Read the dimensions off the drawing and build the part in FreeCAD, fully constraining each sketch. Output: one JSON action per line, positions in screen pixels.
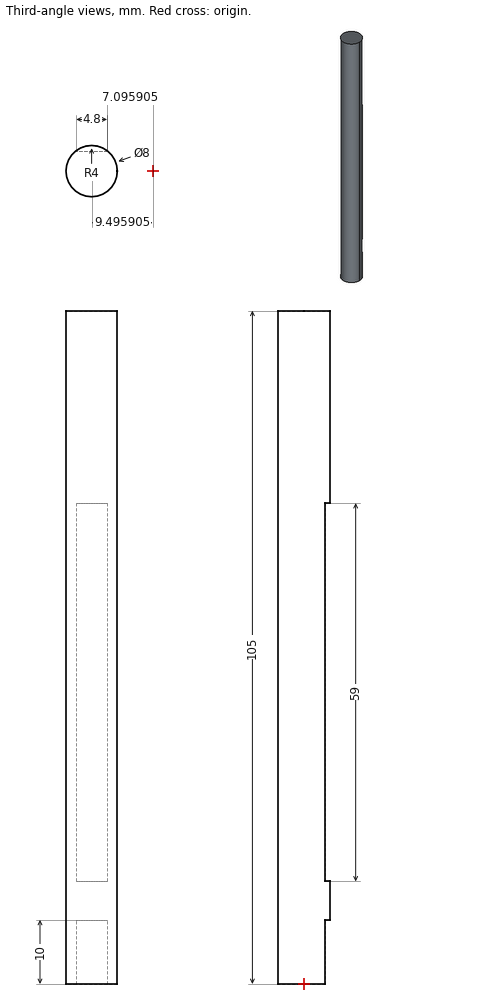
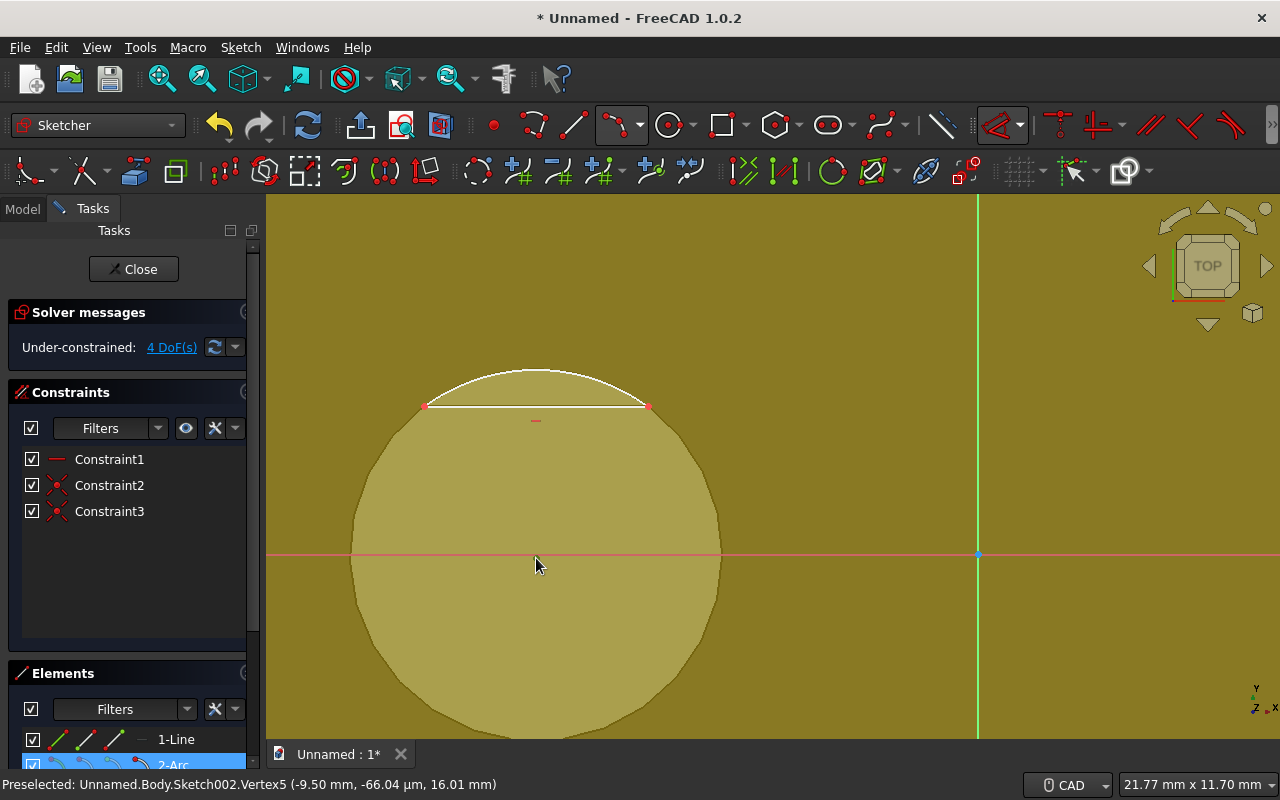
{"action": "left_click", "coordinate": [353, 555]}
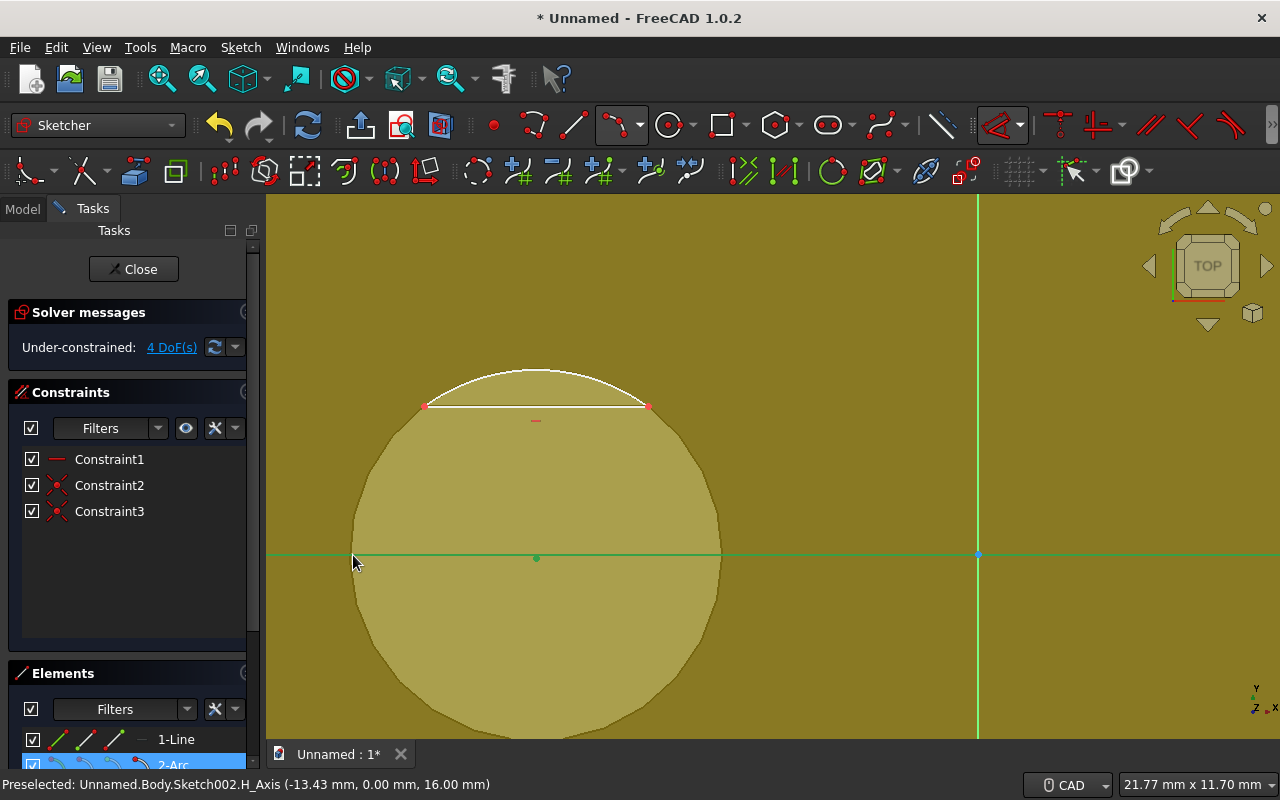
{"action": "key", "text": "c"}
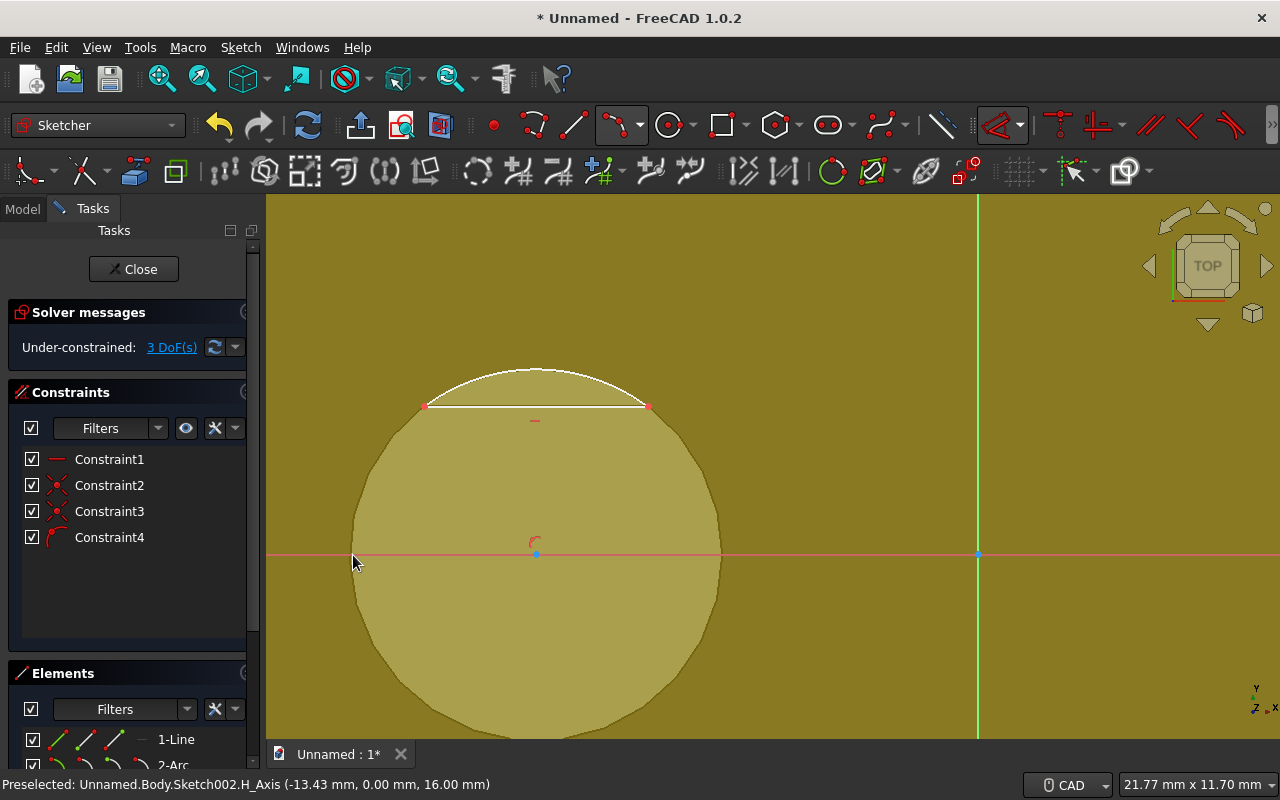
{"action": "left_click", "coordinate": [584, 376]}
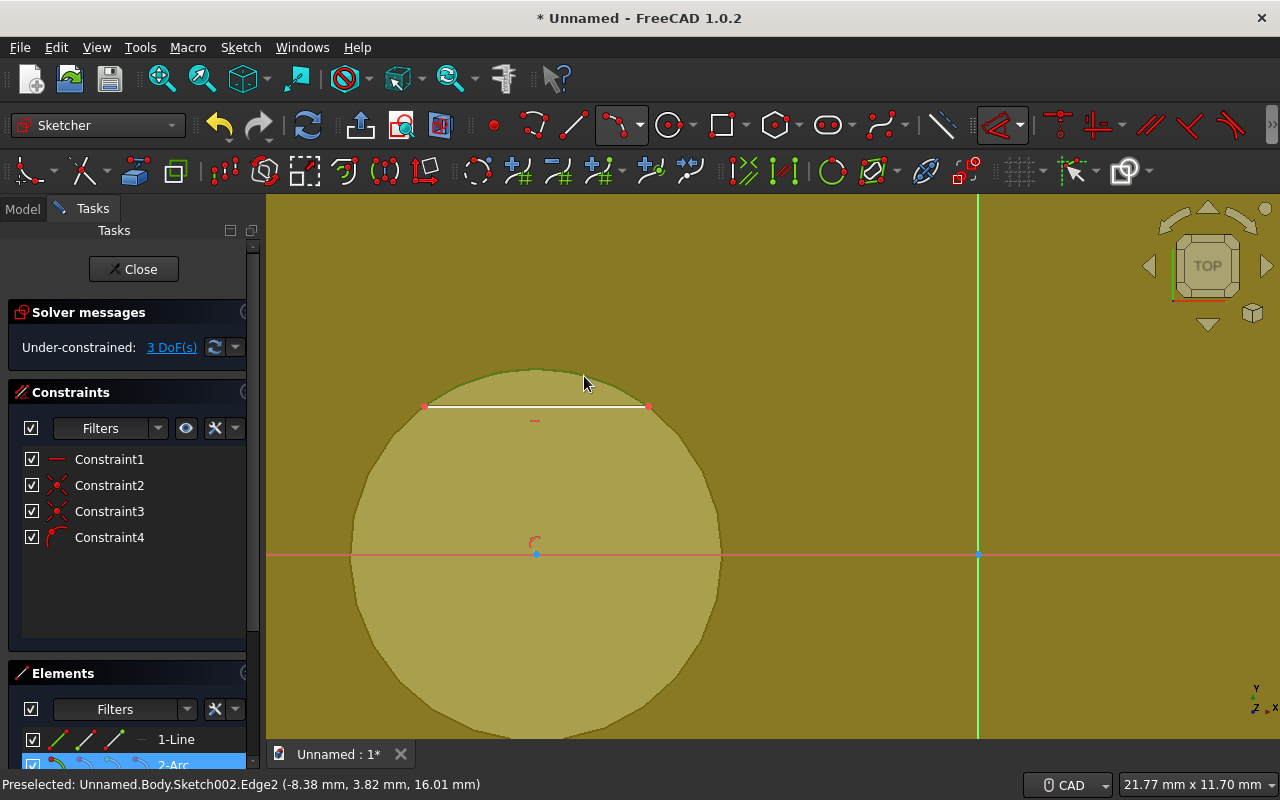
{"action": "left_click", "coordinate": [1022, 126]}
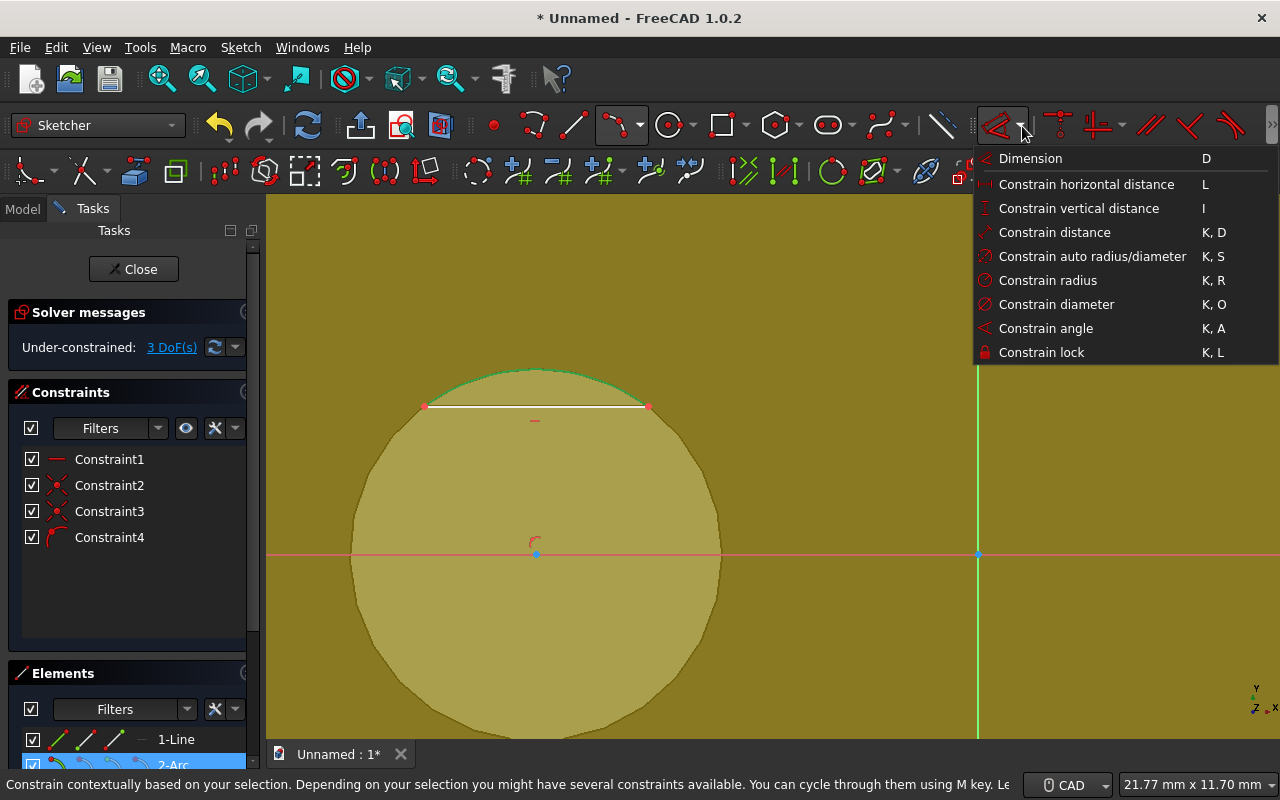
{"action": "left_click", "coordinate": [1126, 280]}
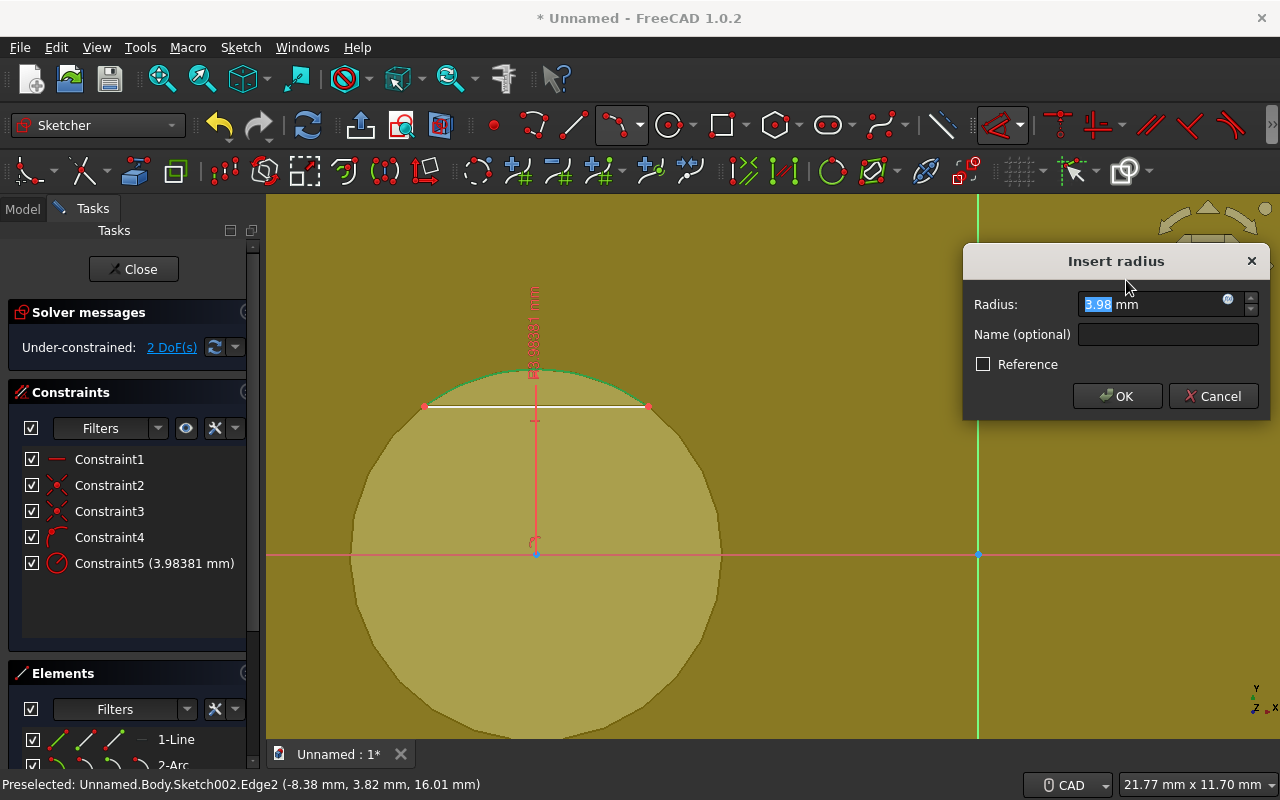
{"action": "type", "text": "4"}
{"action": "key", "text": "Return"}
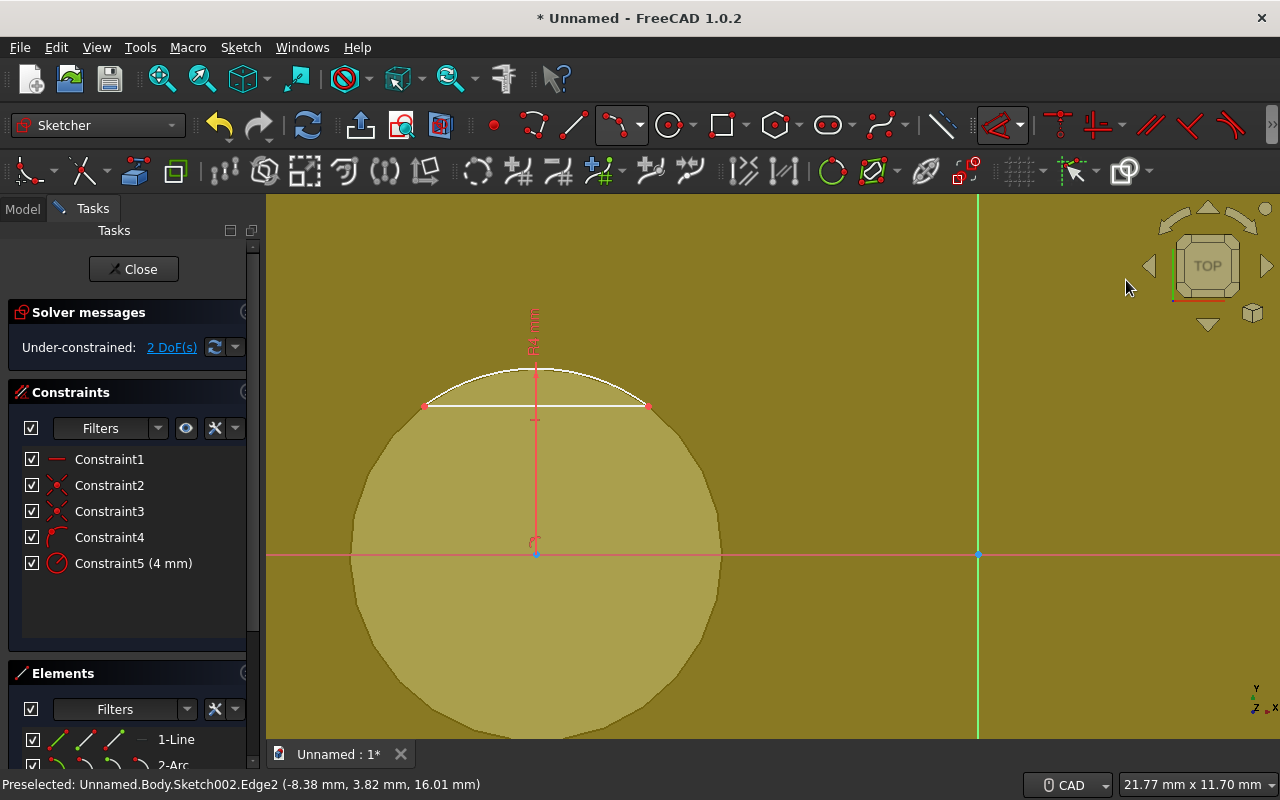
{"action": "left_click", "coordinate": [581, 406]}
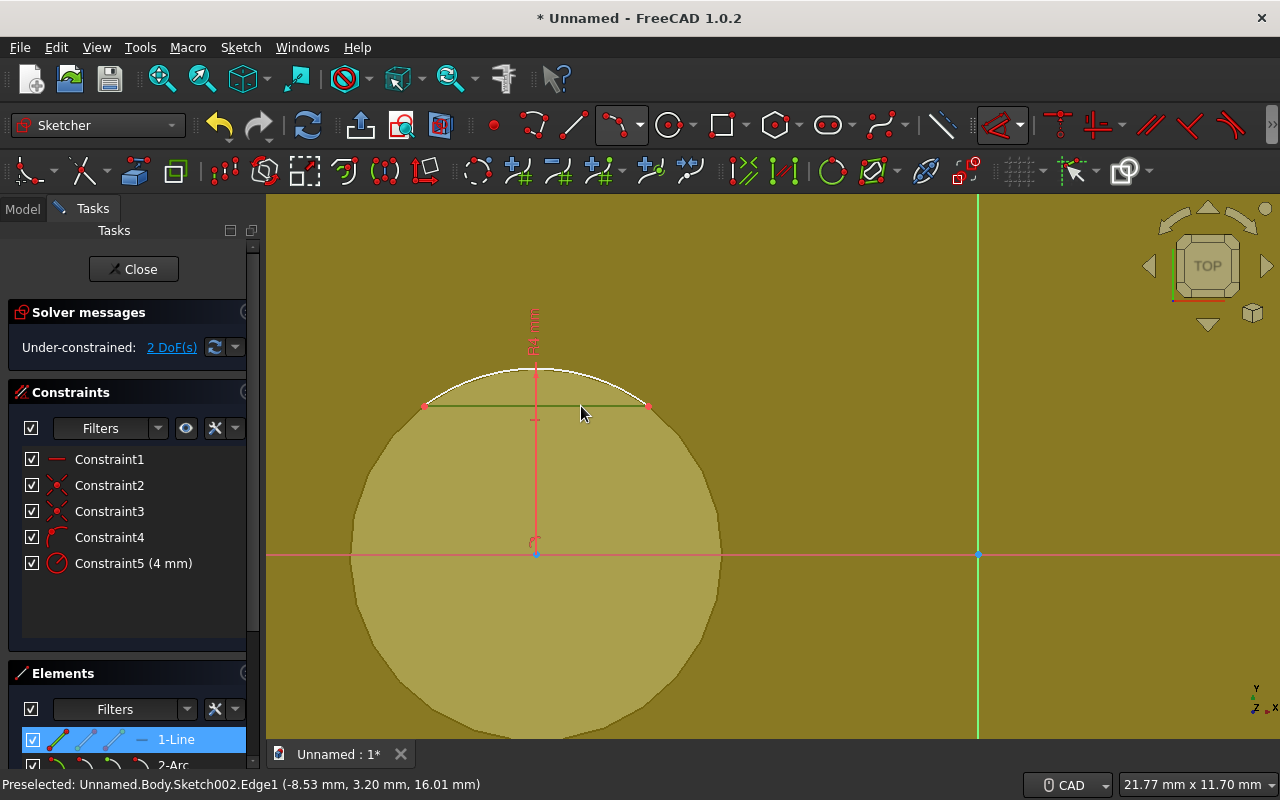
{"action": "key", "text": "l"}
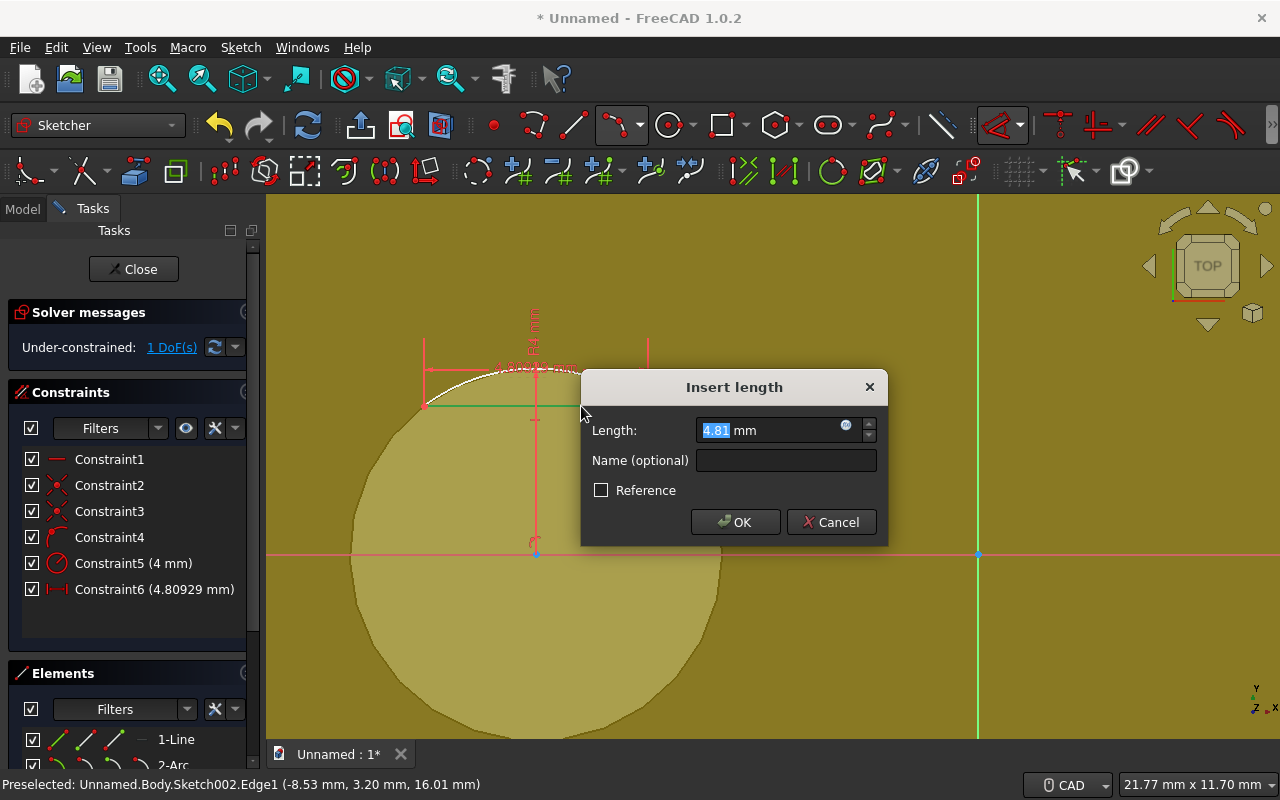
{"action": "type", "text": "4.8"}
{"action": "key", "text": "Return"}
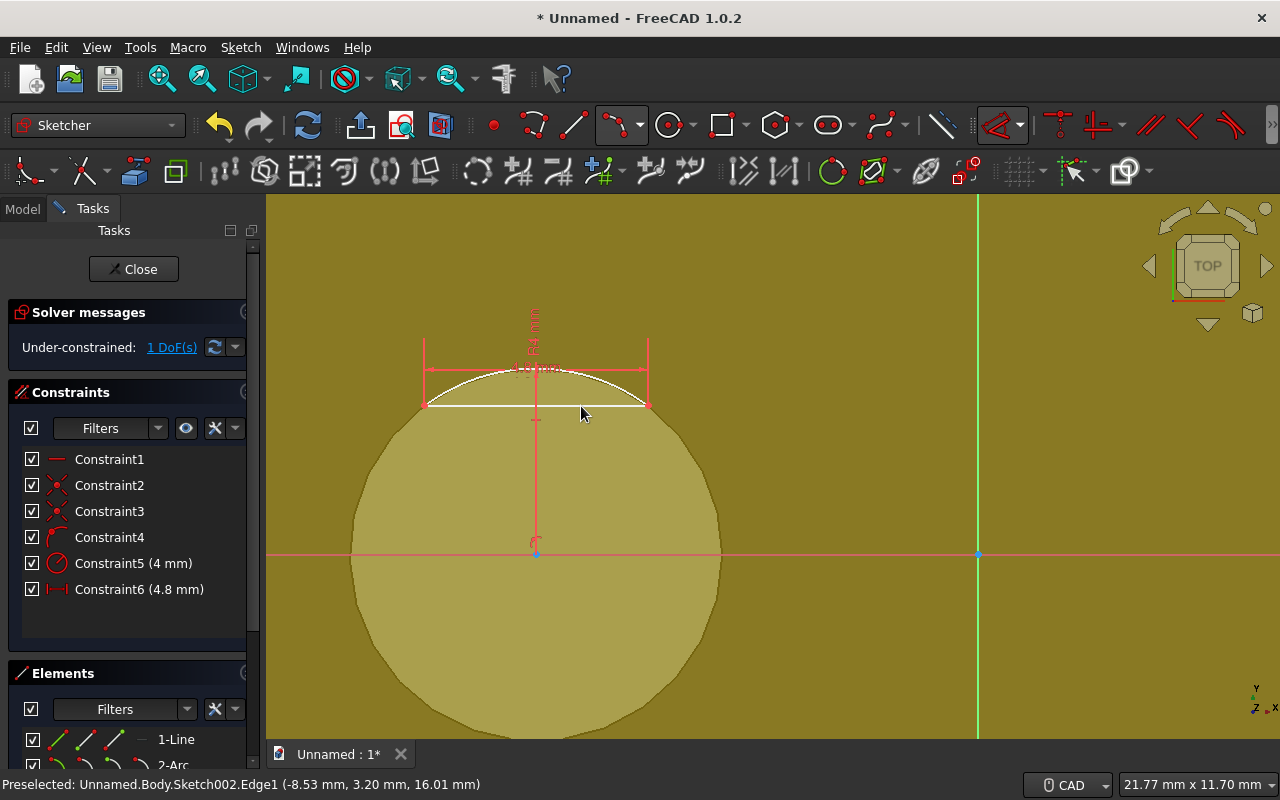
{"action": "left_click", "coordinate": [648, 406]}